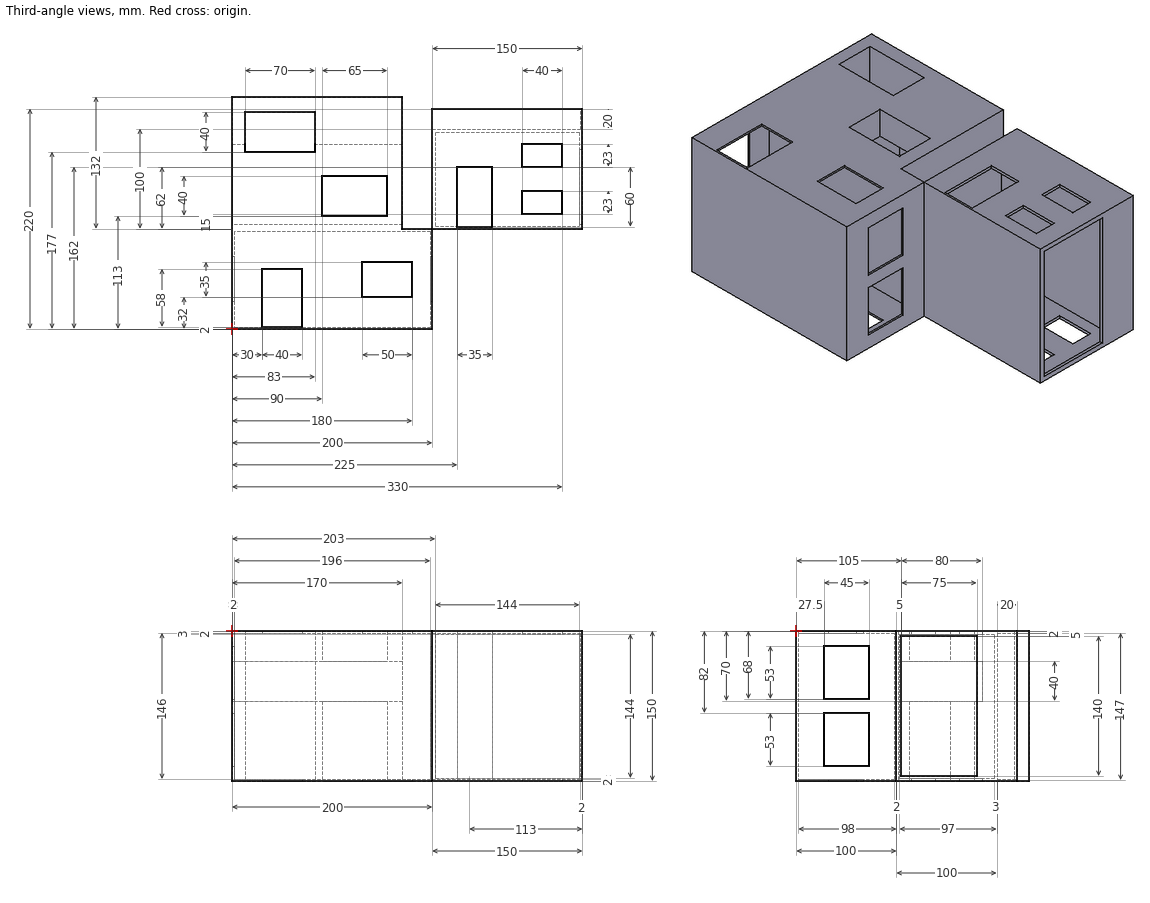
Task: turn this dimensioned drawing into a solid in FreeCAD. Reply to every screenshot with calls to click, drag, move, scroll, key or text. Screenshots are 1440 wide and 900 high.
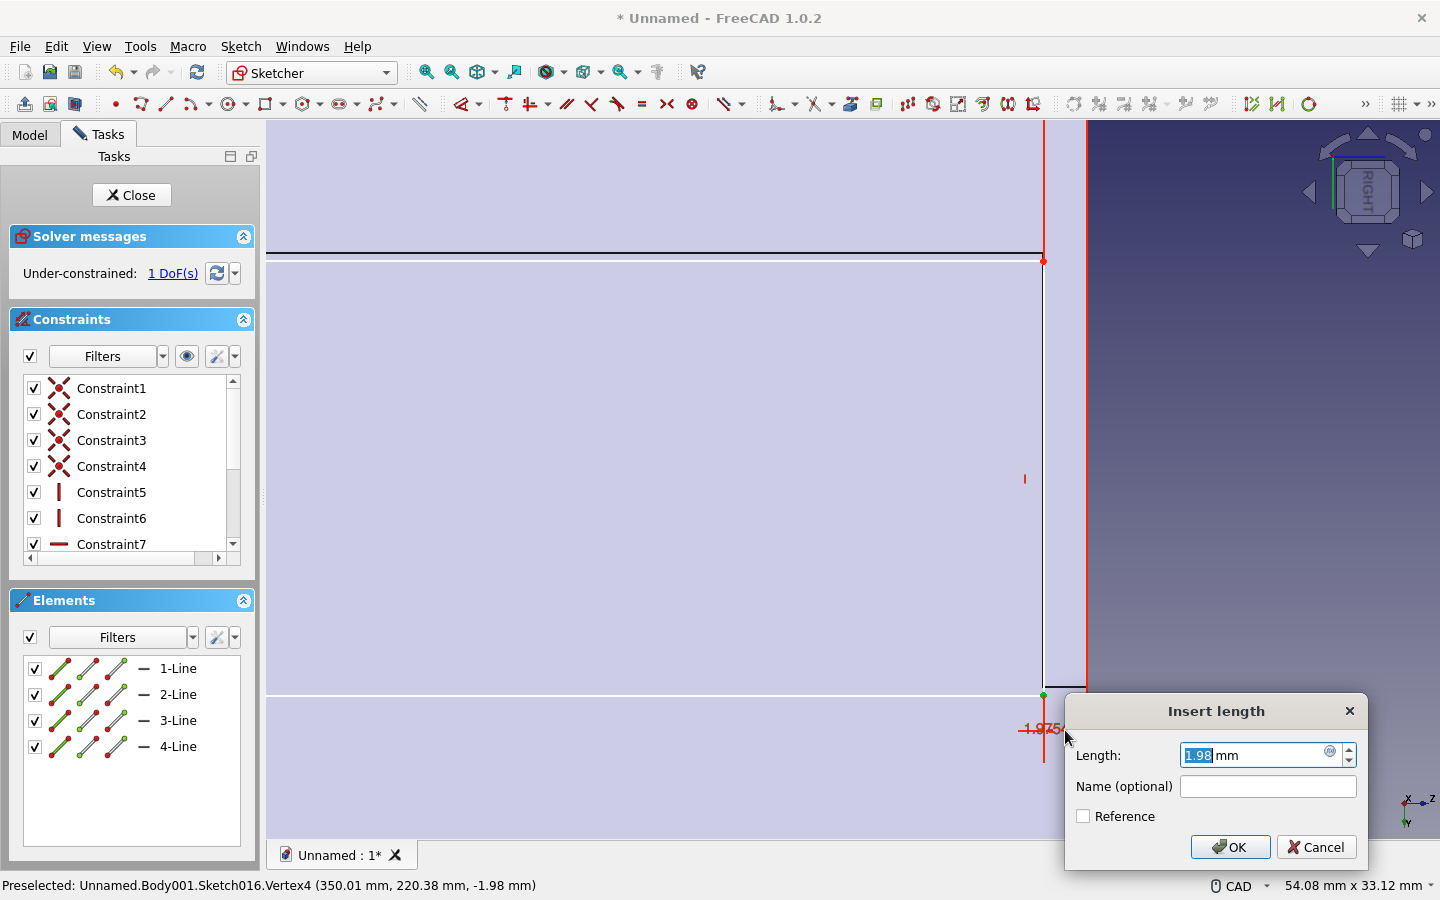
text(2)
key(Return)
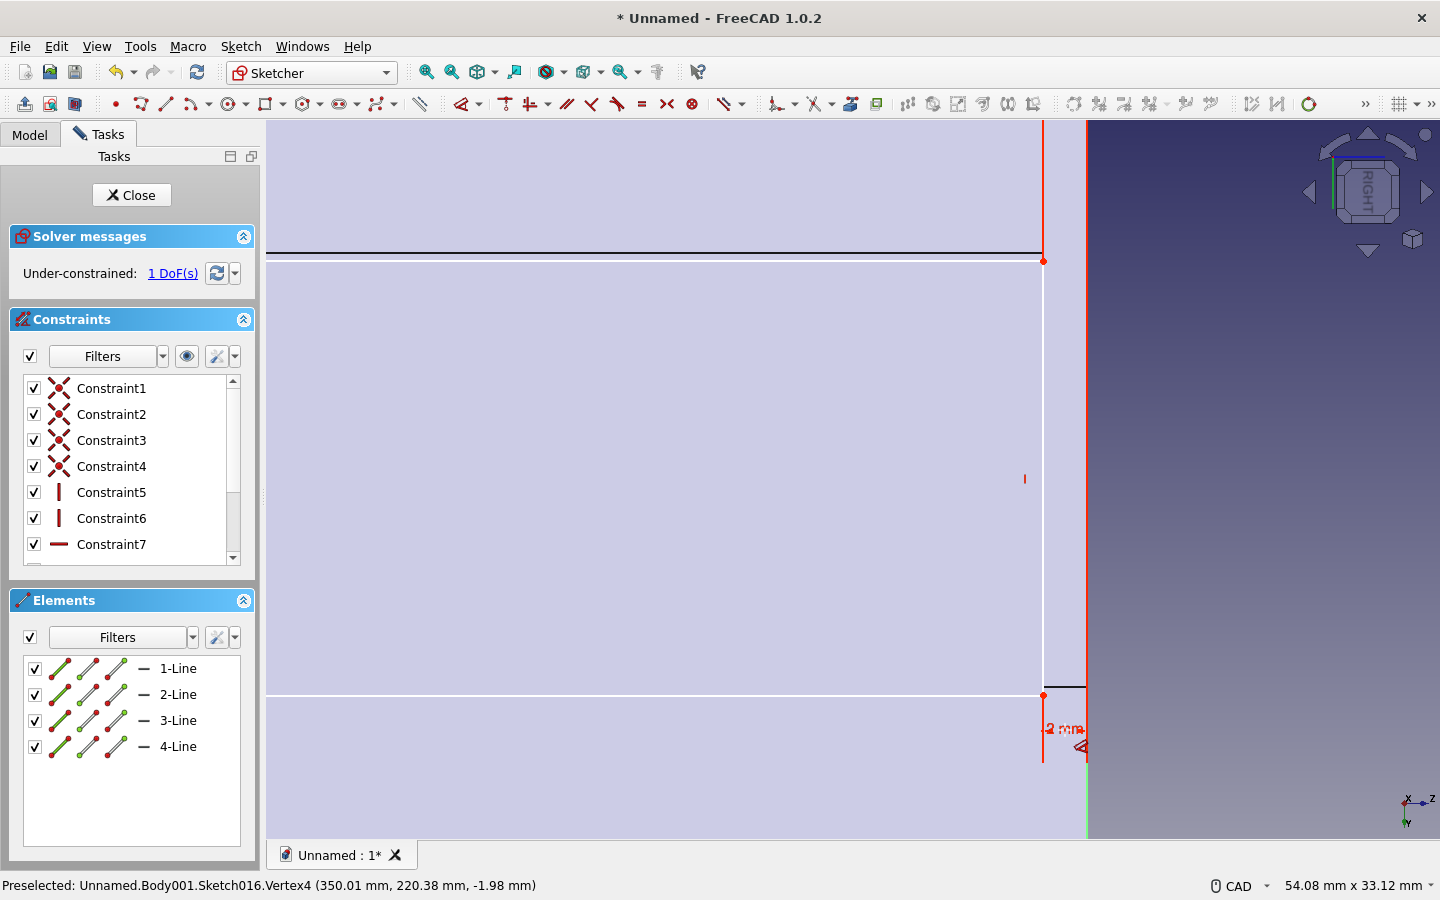
scroll(1045, 696, down, 9)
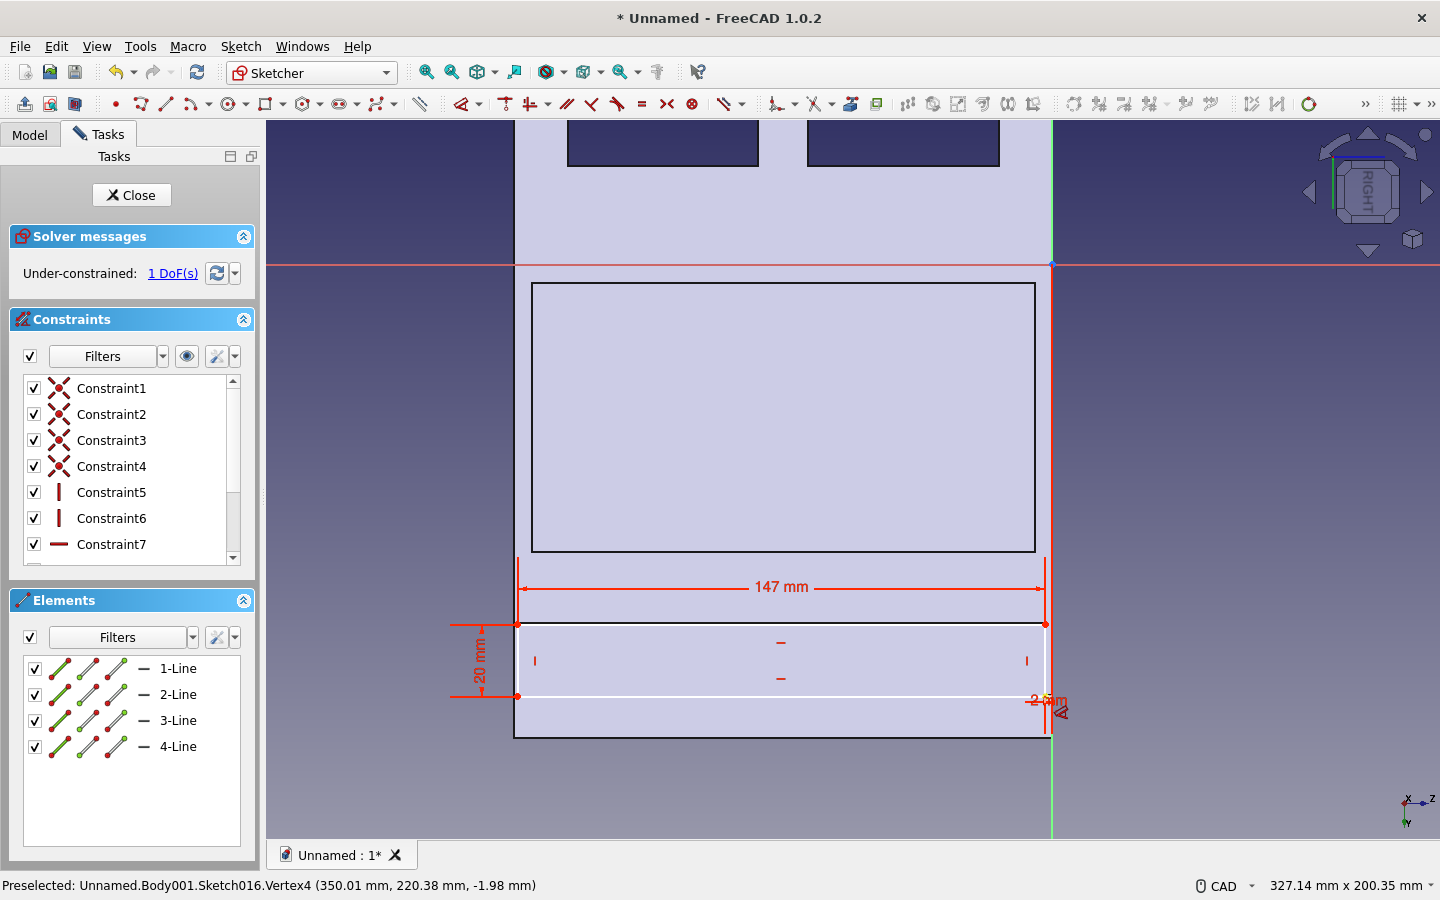
click(518, 625)
click(1086, 445)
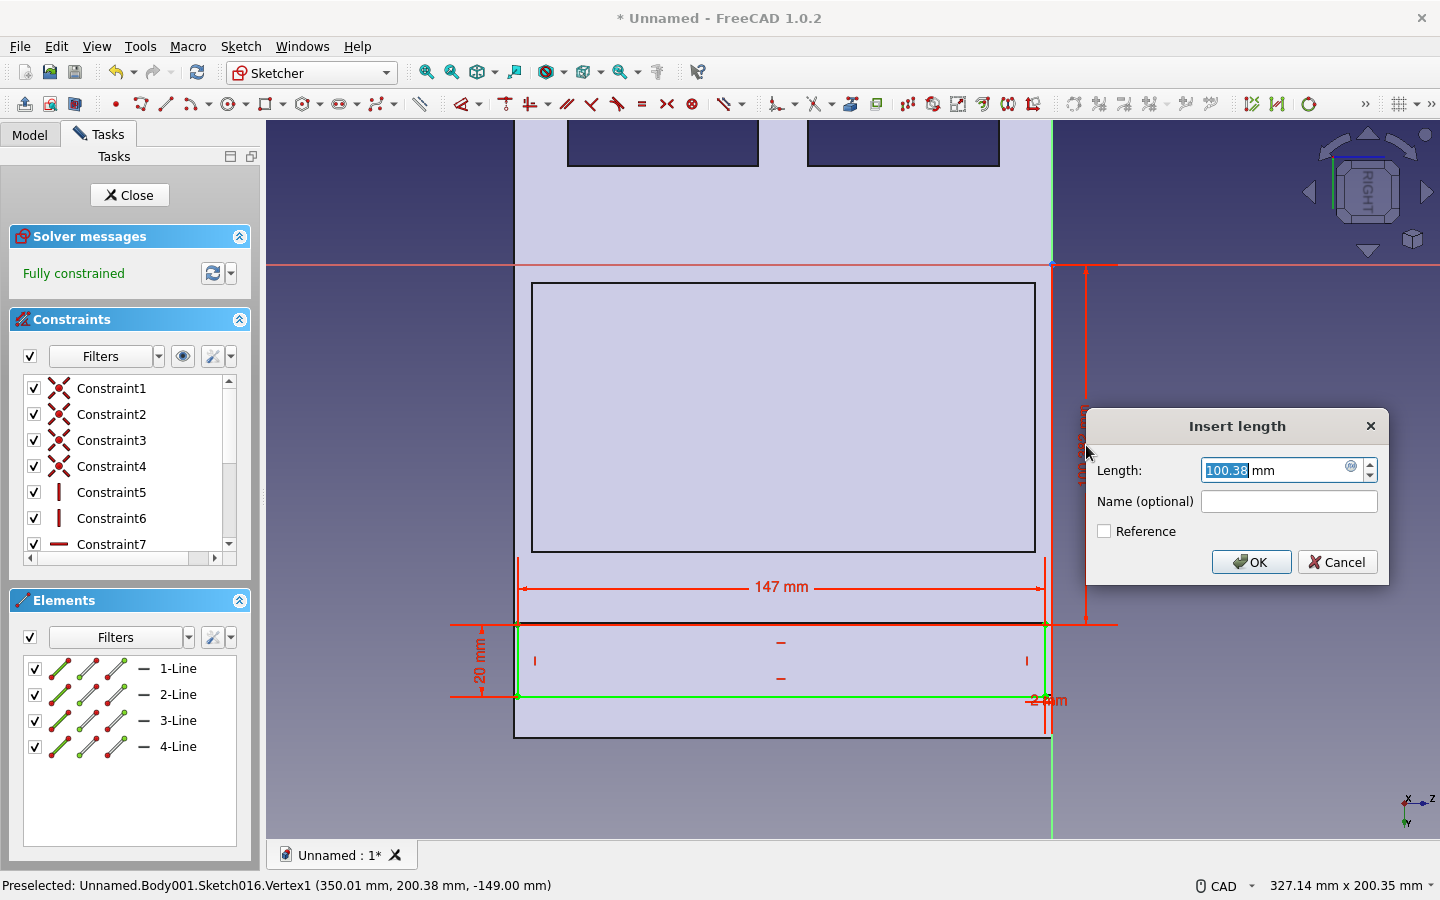
text(100)
key(Return)
key(Escape)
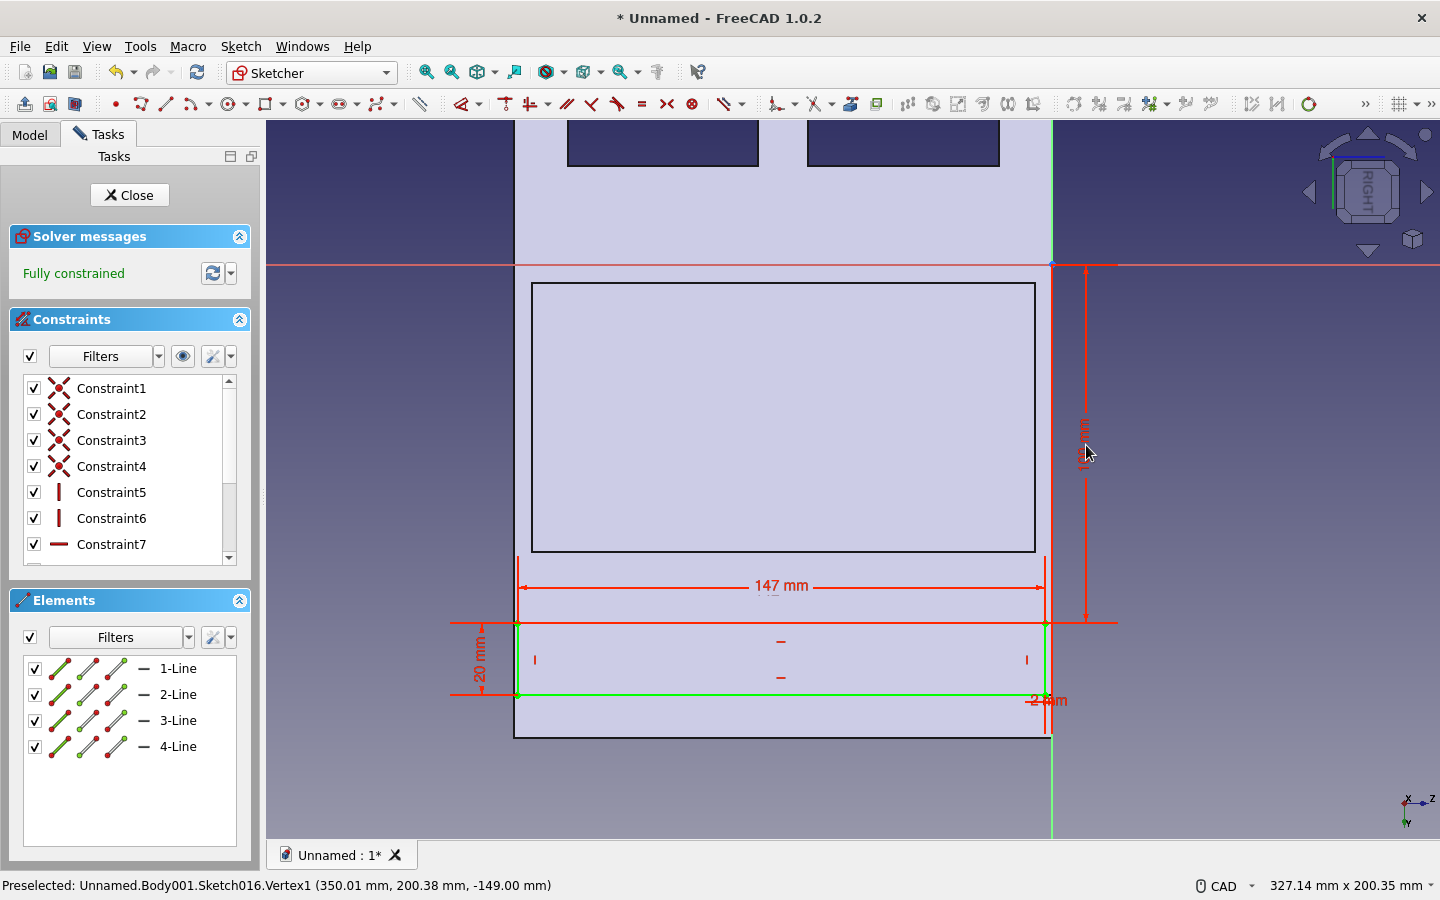
click(130, 195)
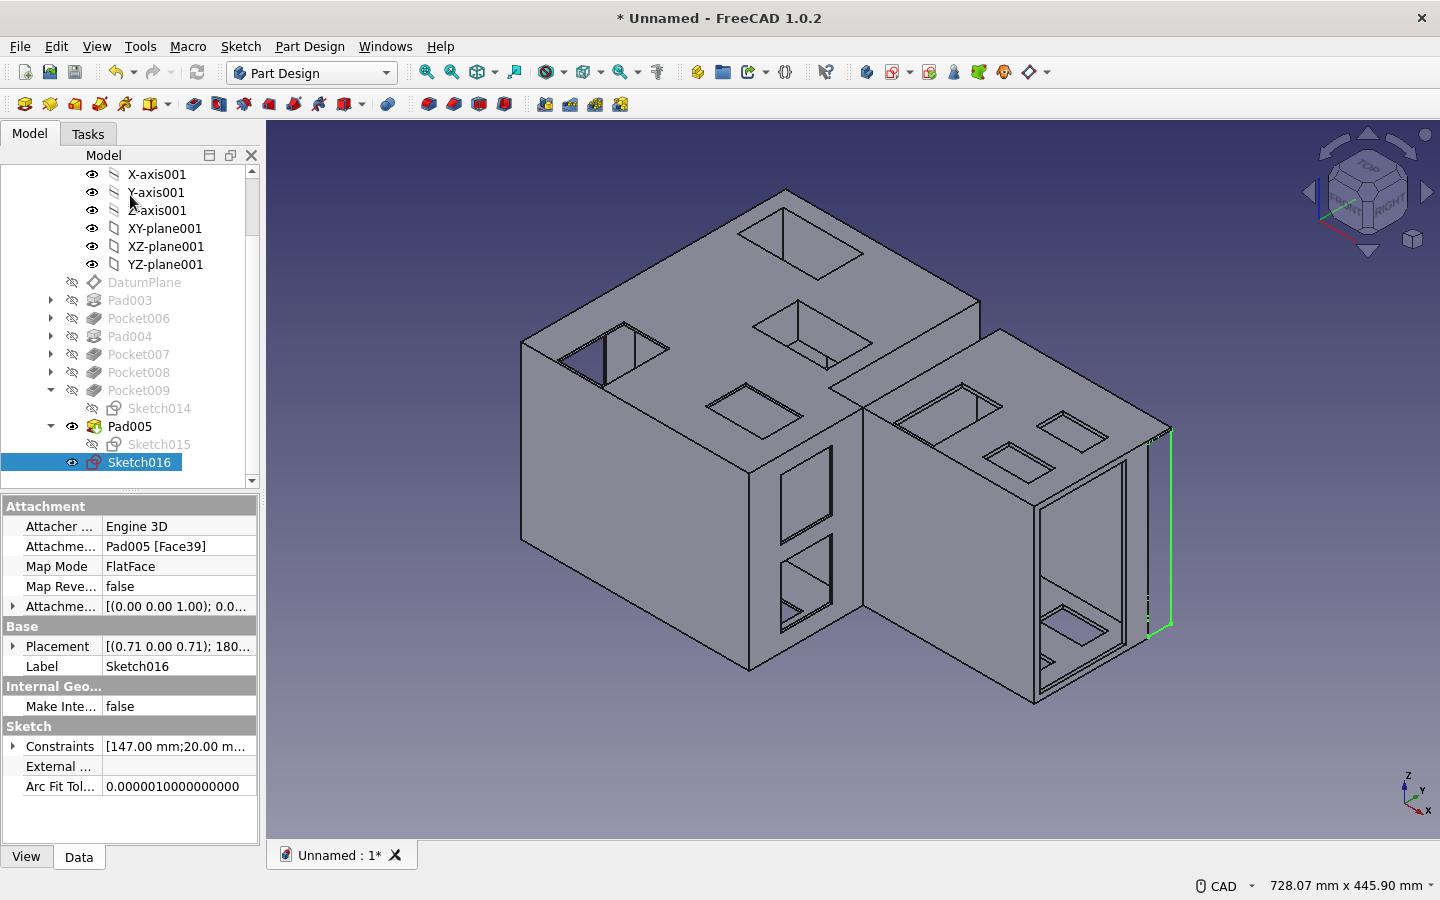
click(25, 104)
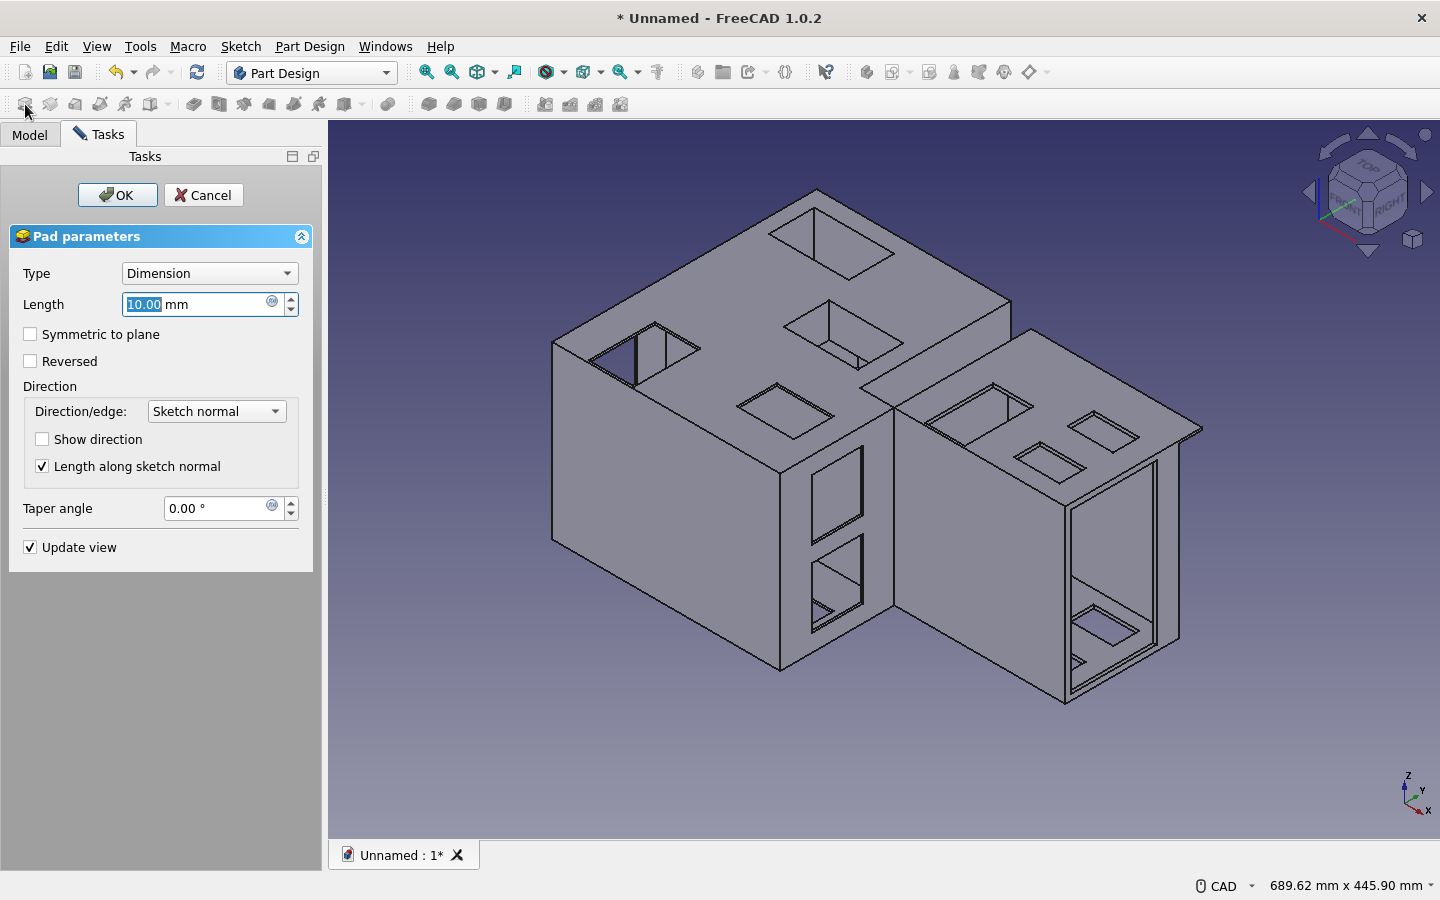
text(2)
key(Tab)